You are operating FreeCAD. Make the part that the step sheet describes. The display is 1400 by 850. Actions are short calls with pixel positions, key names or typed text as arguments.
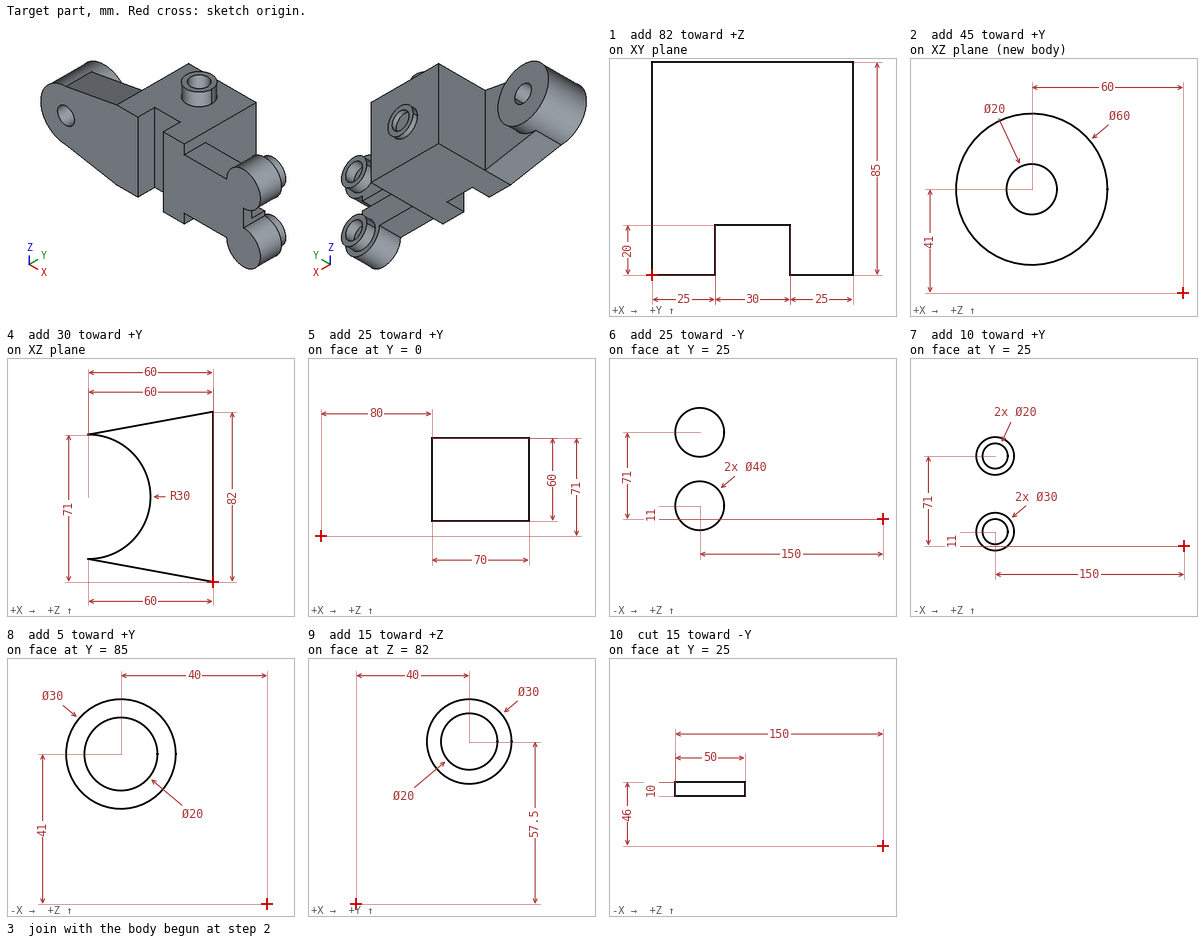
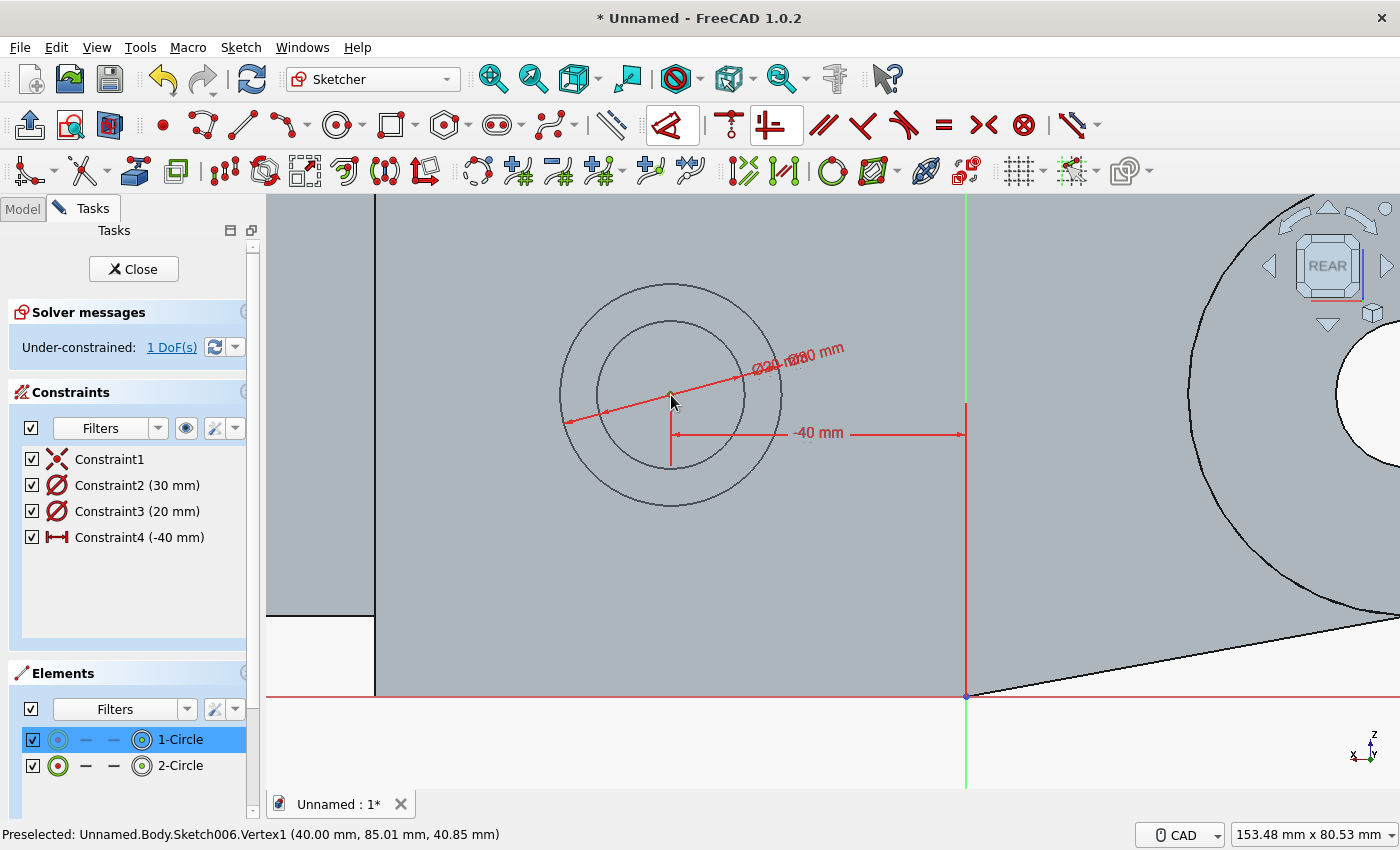
key(i)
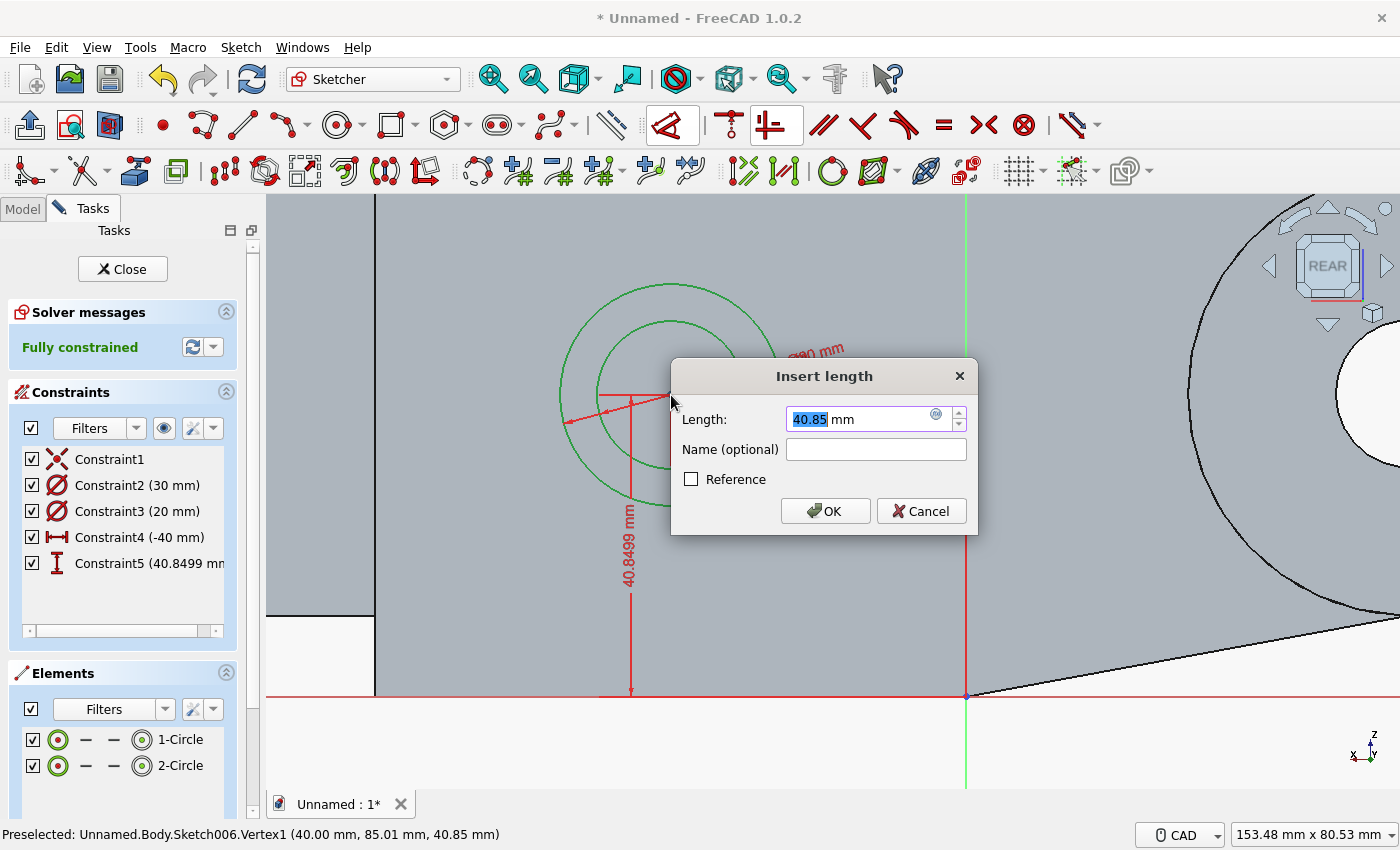
text(41)
key(Return)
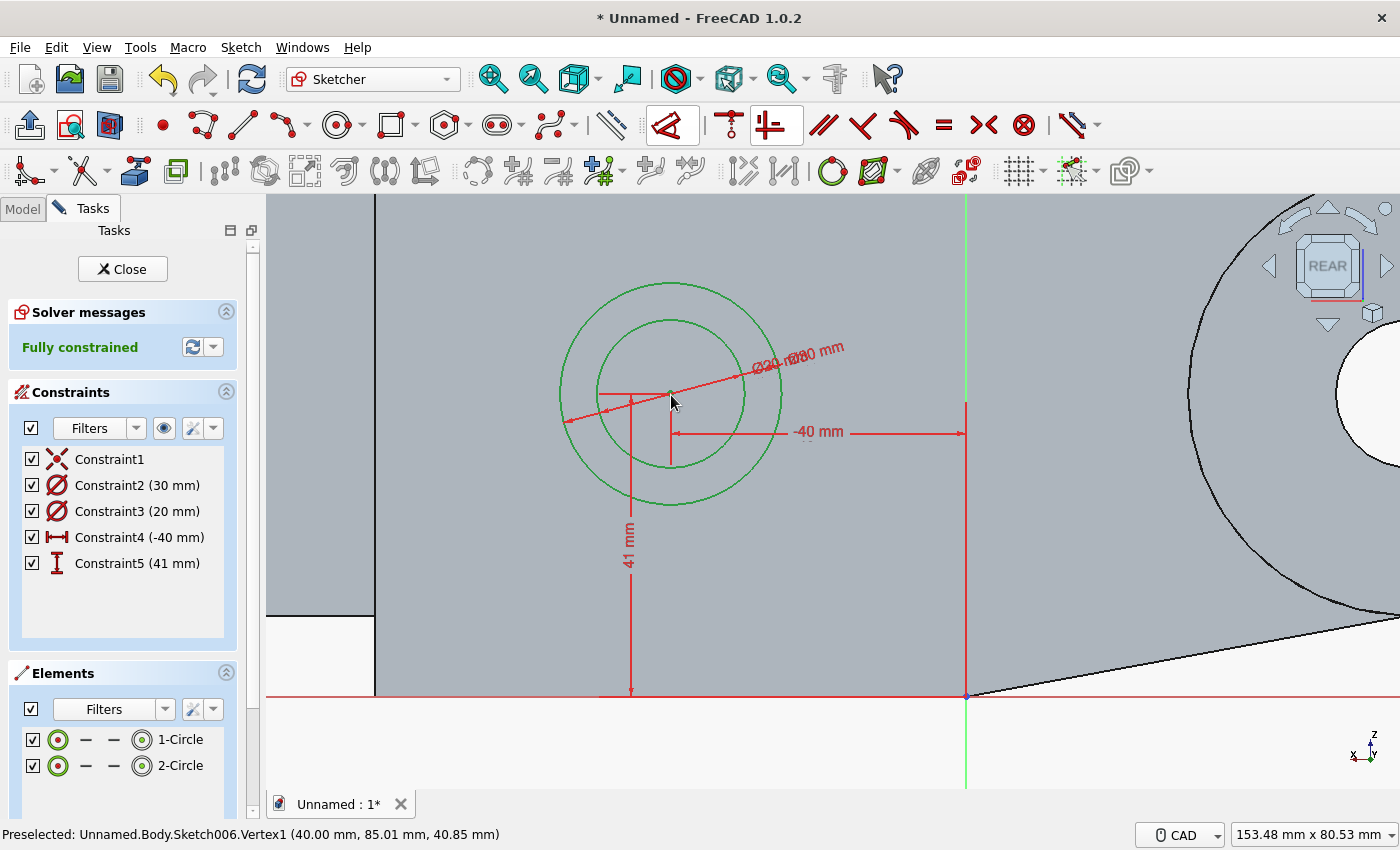
click(123, 269)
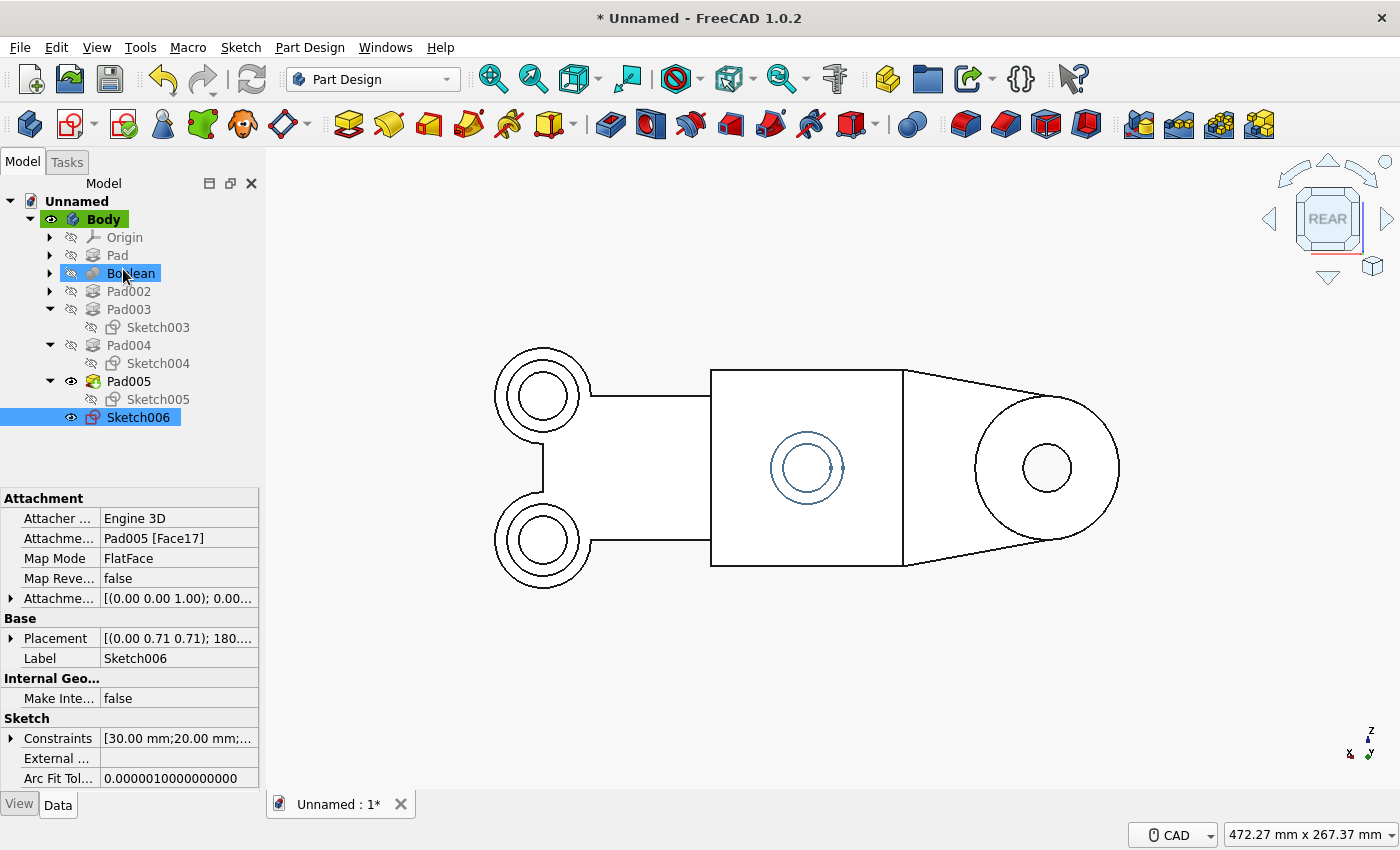
click(350, 124)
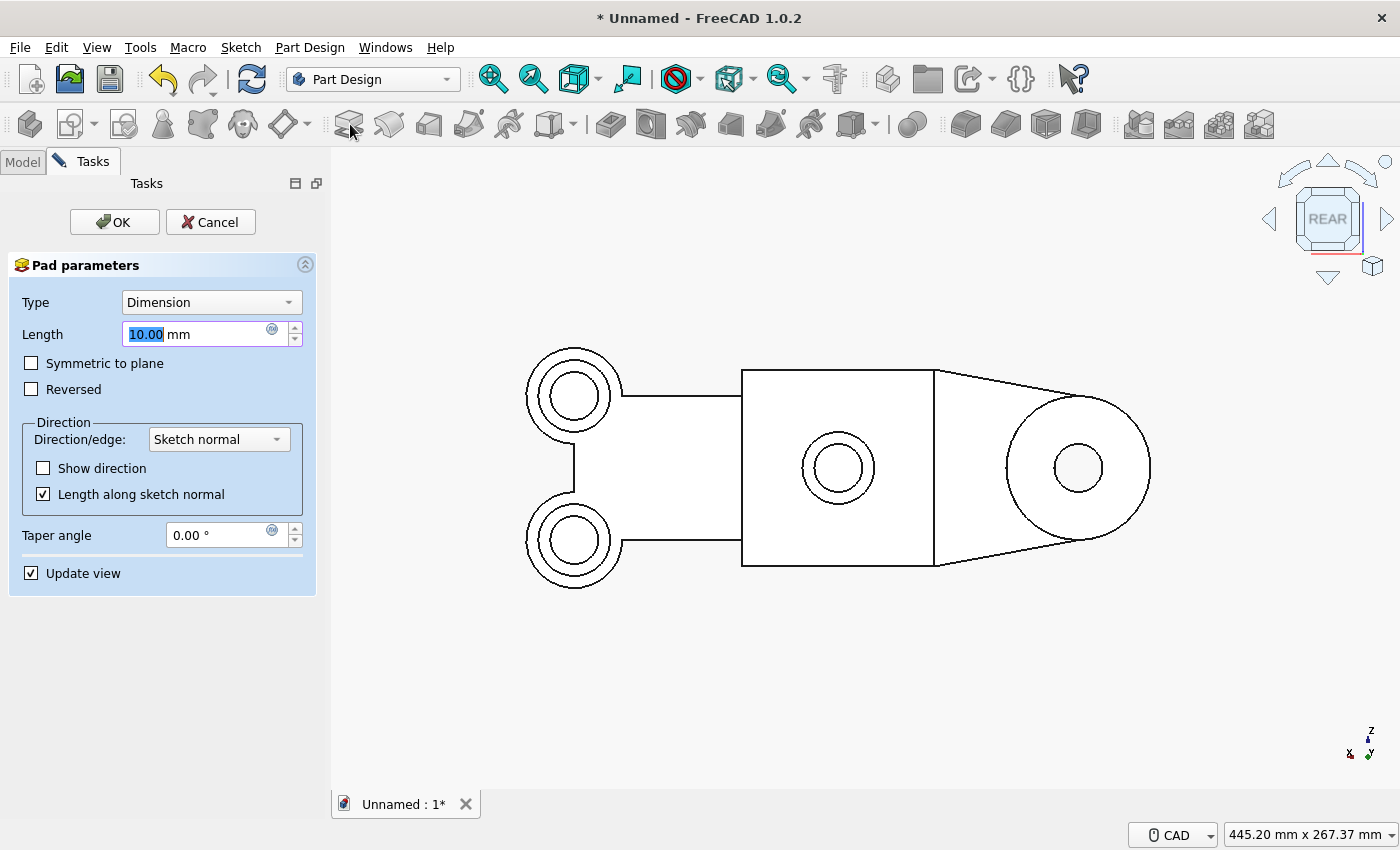
text(5)
key(Tab)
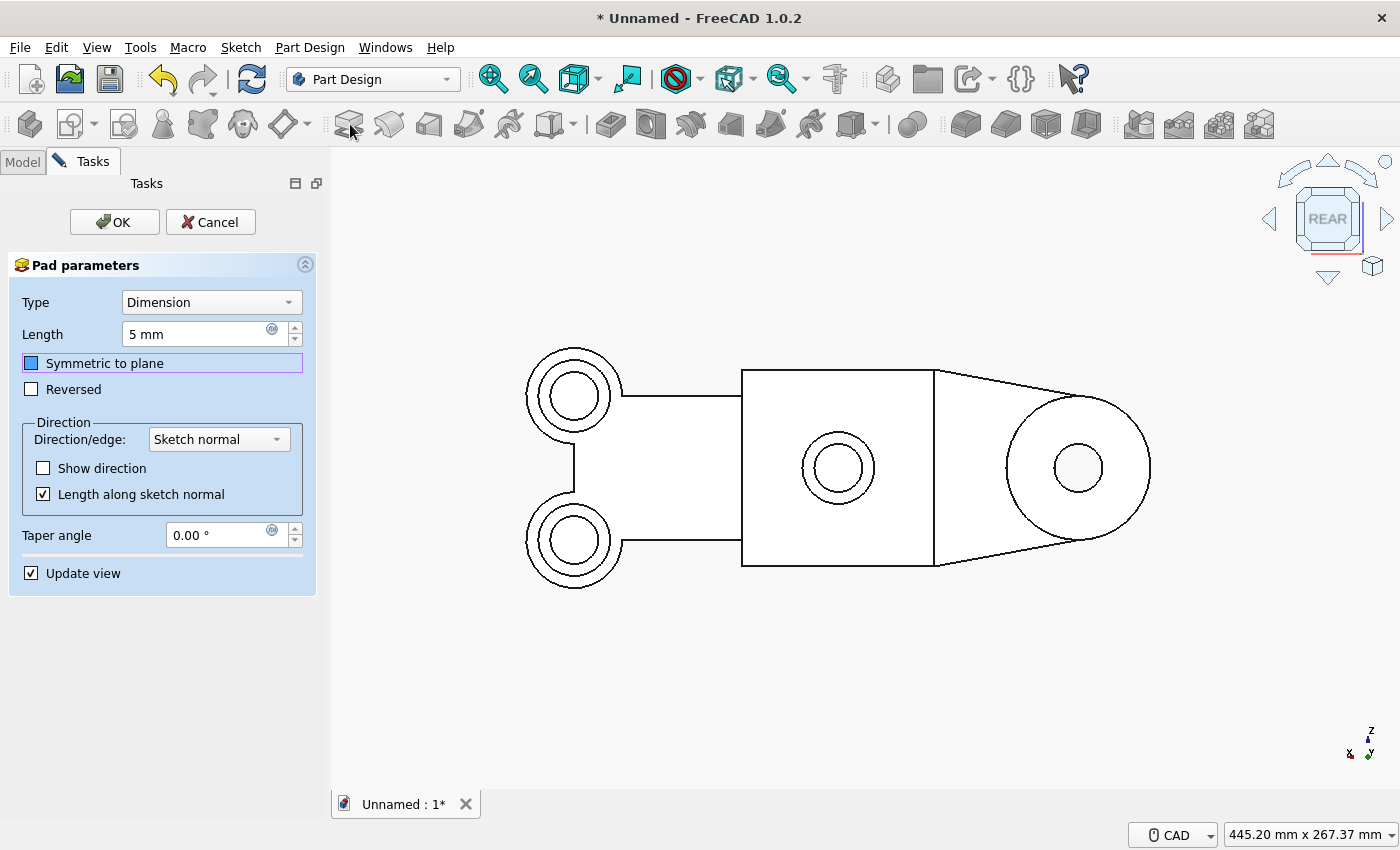
click(115, 222)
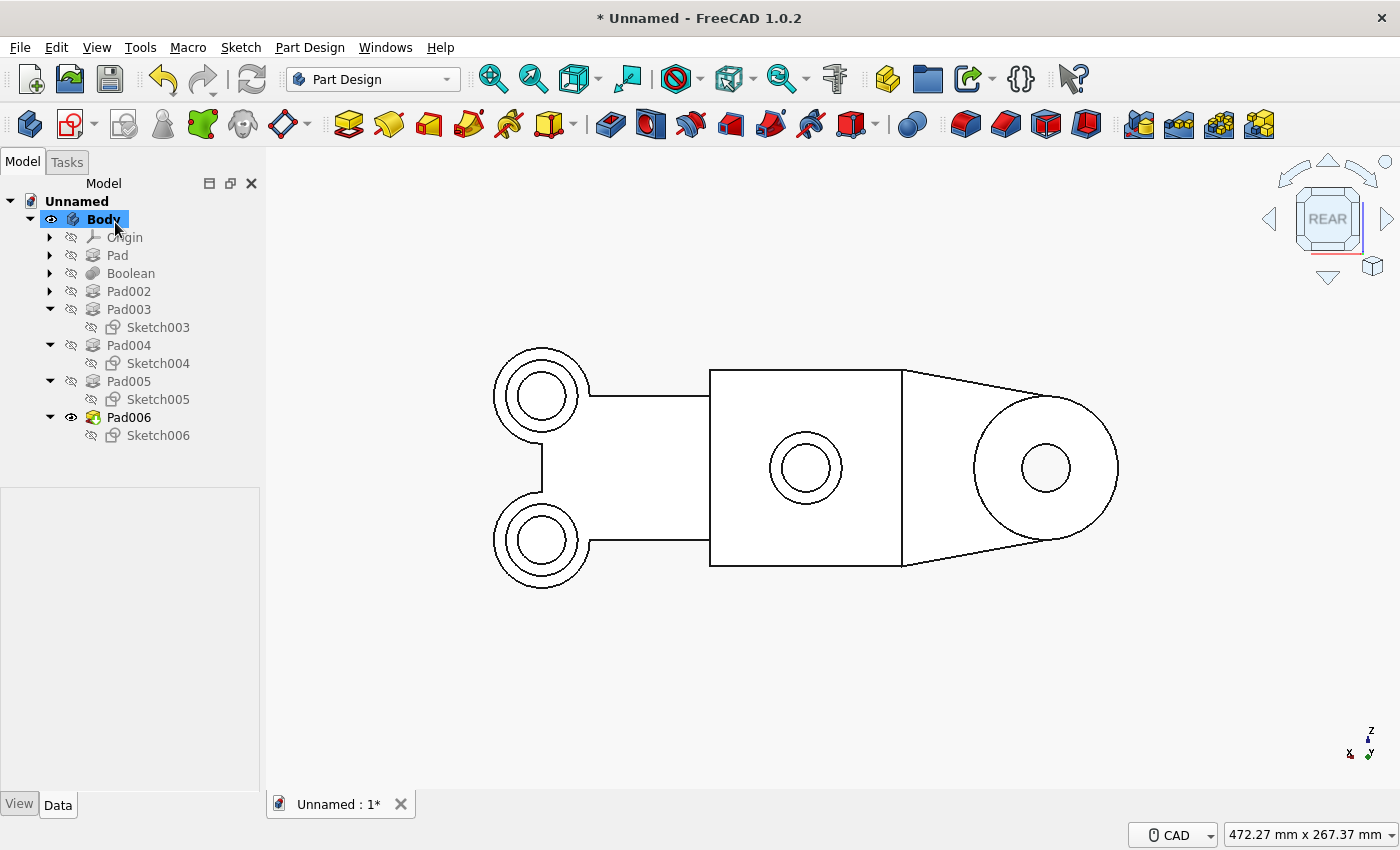
key(0)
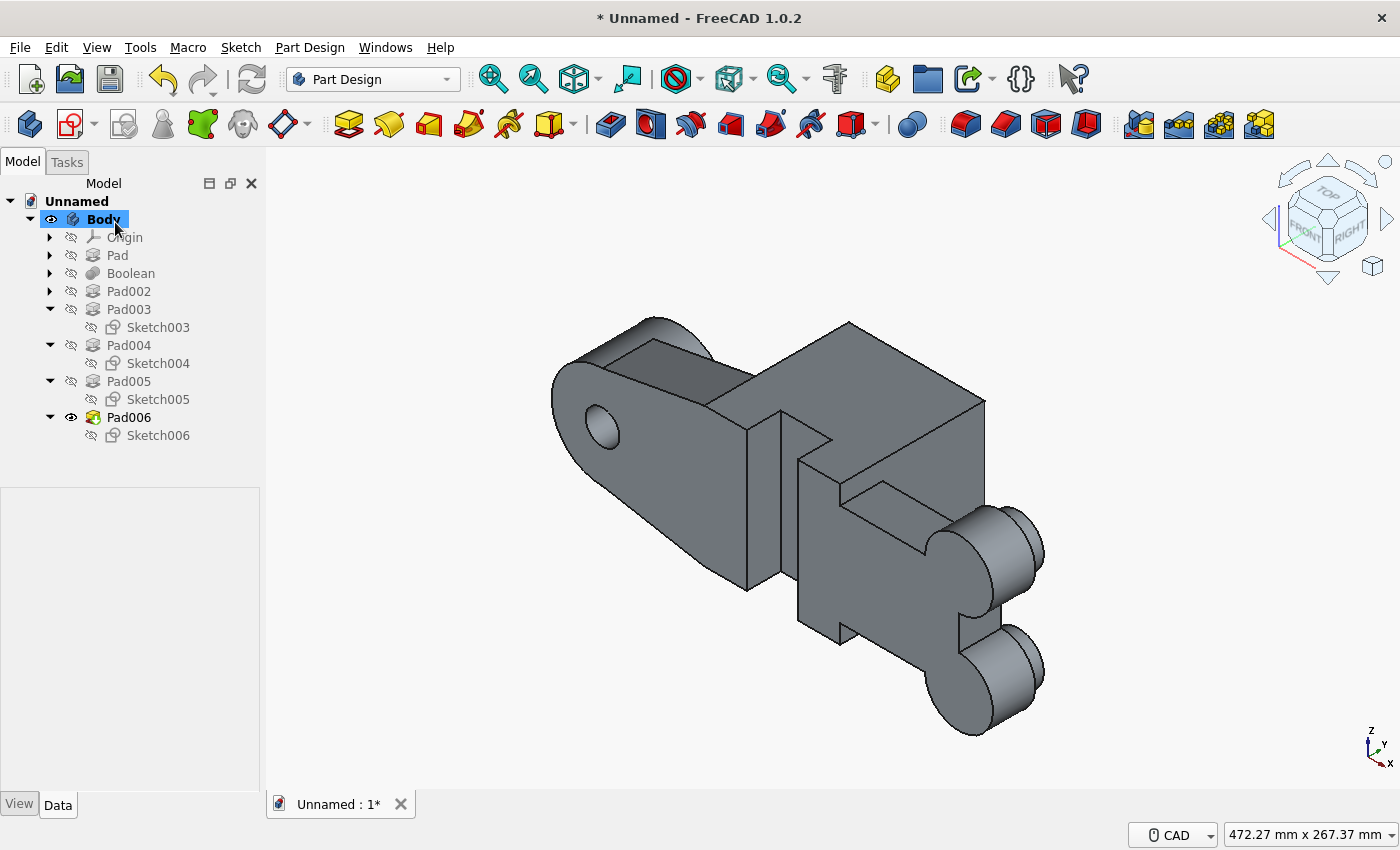
click(865, 390)